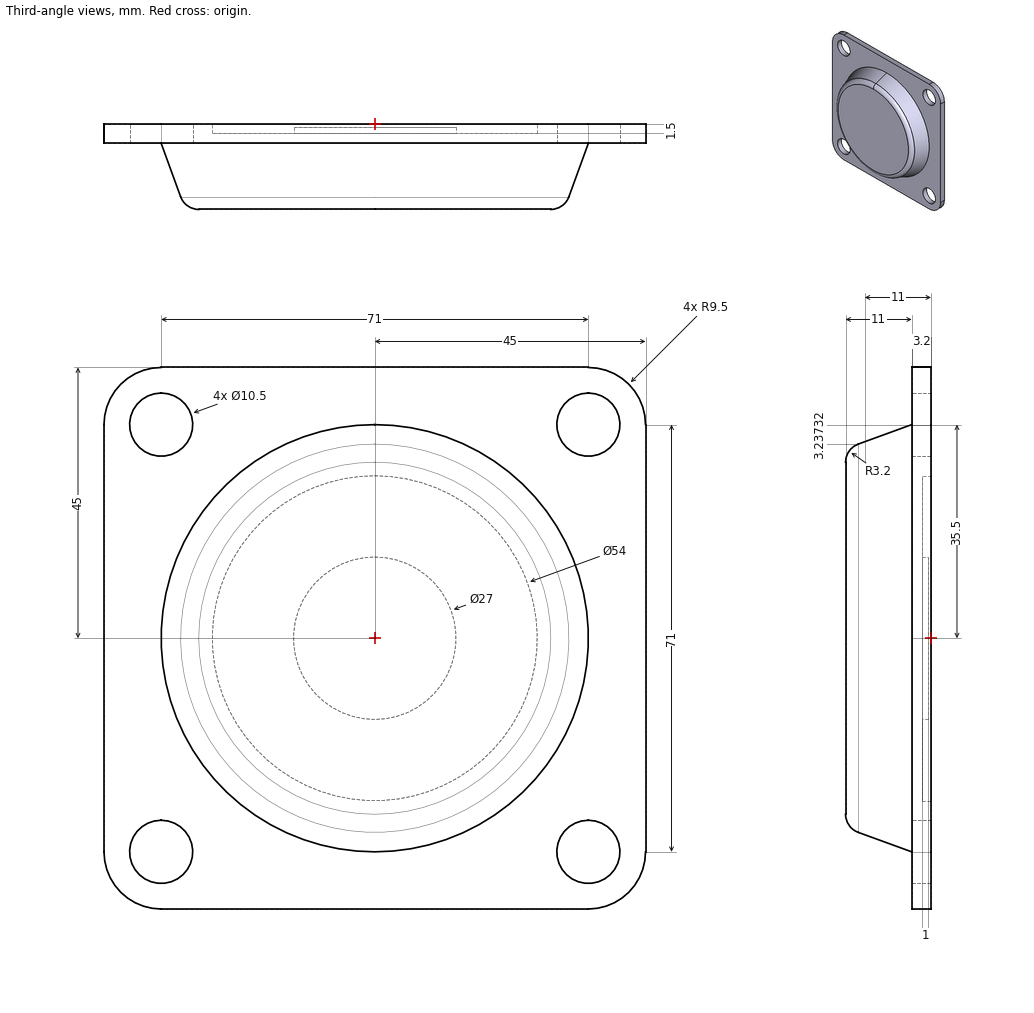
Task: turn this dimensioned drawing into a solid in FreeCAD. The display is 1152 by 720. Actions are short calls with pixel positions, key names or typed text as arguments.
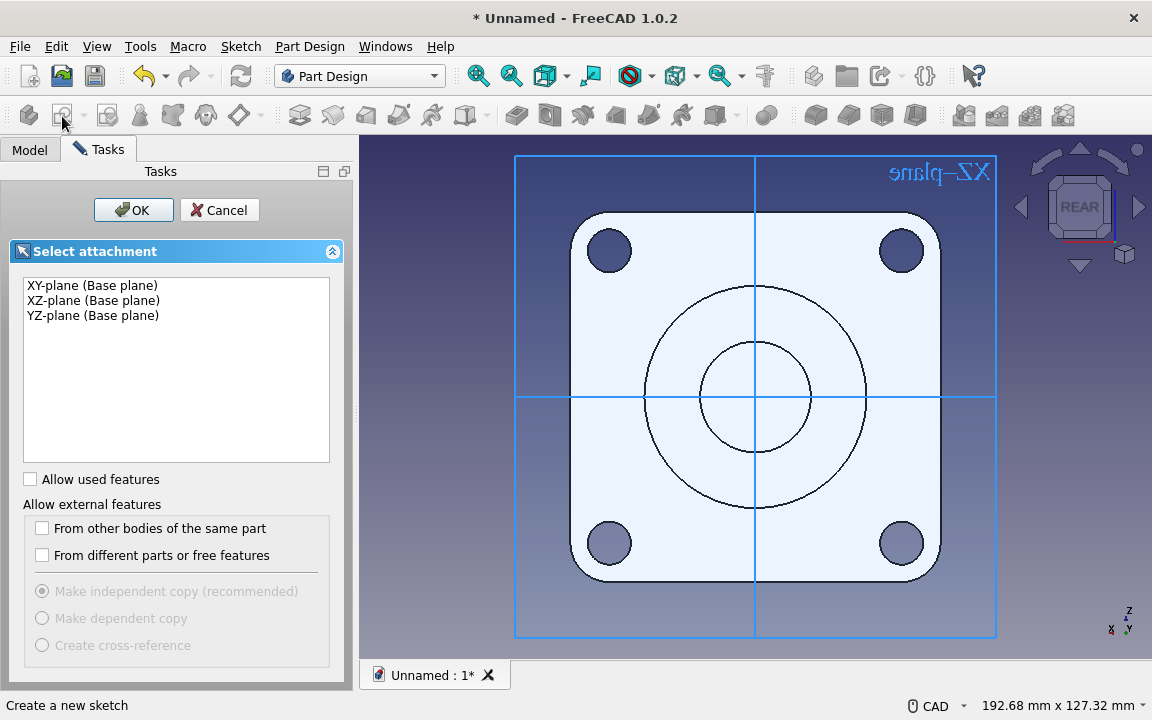
click(84, 316)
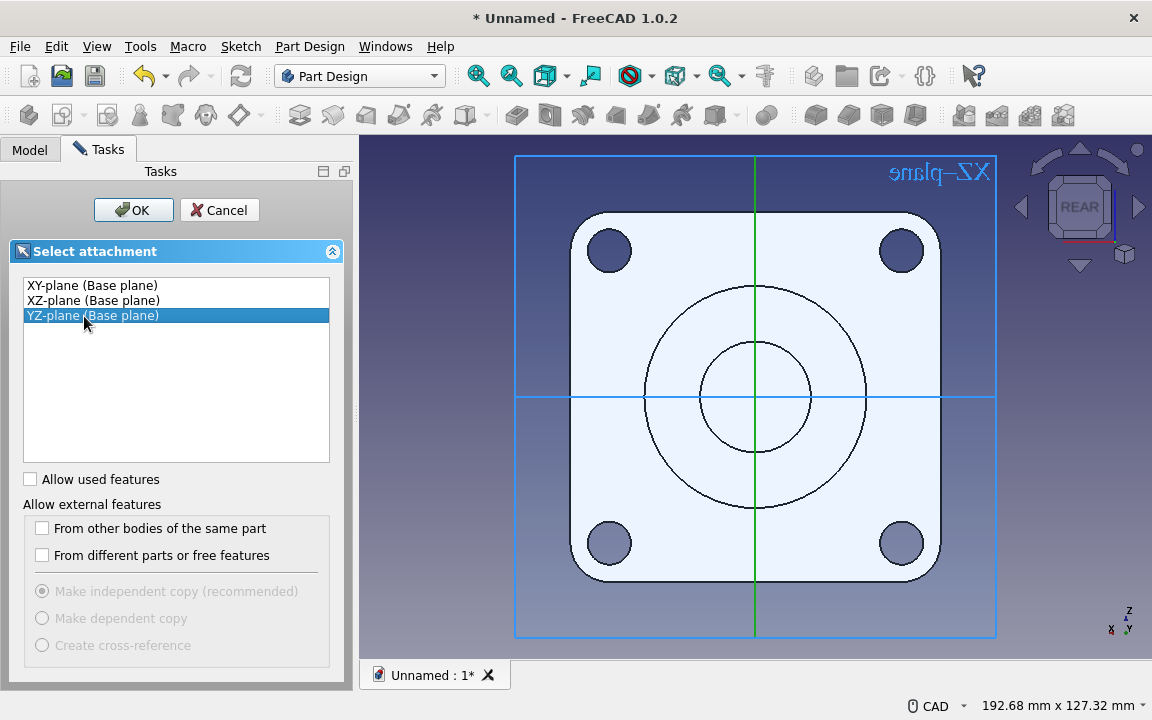
click(134, 210)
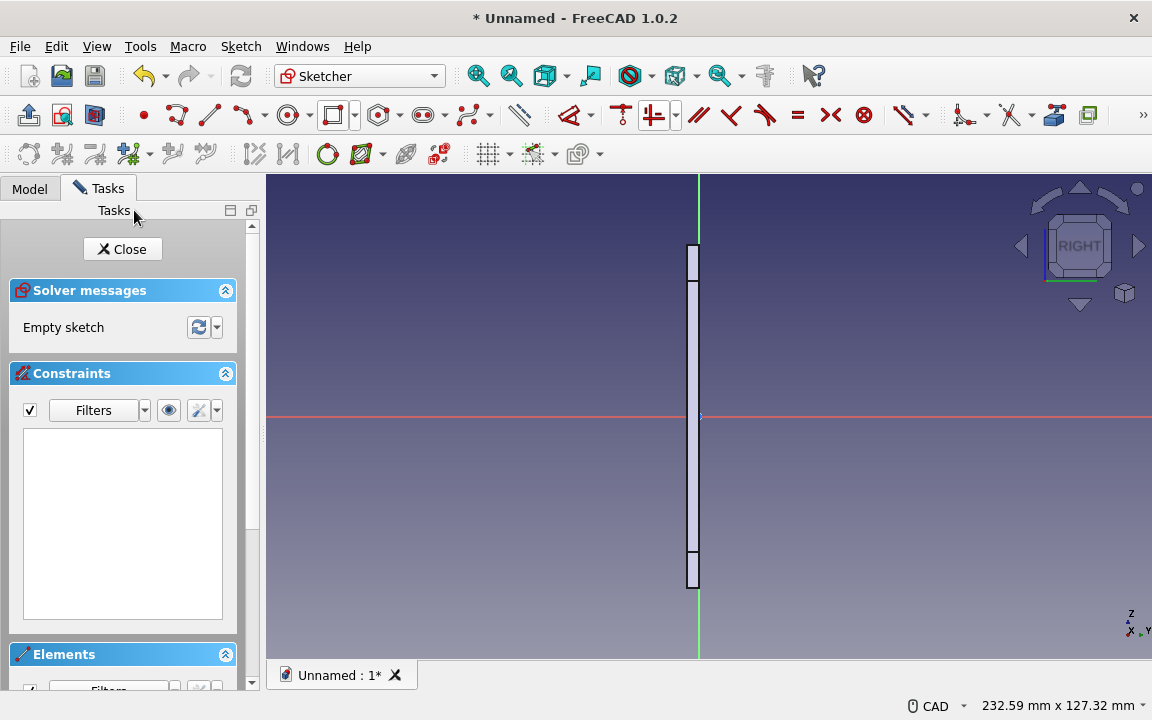
click(95, 116)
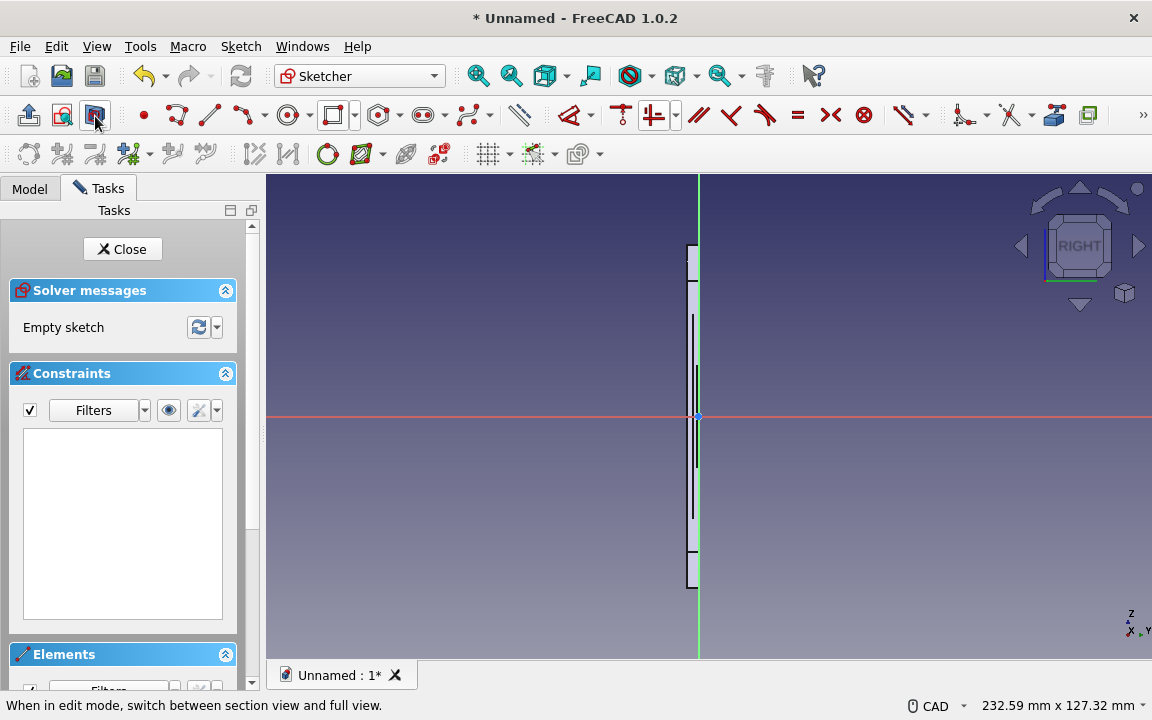
scroll(697, 294, up, 4)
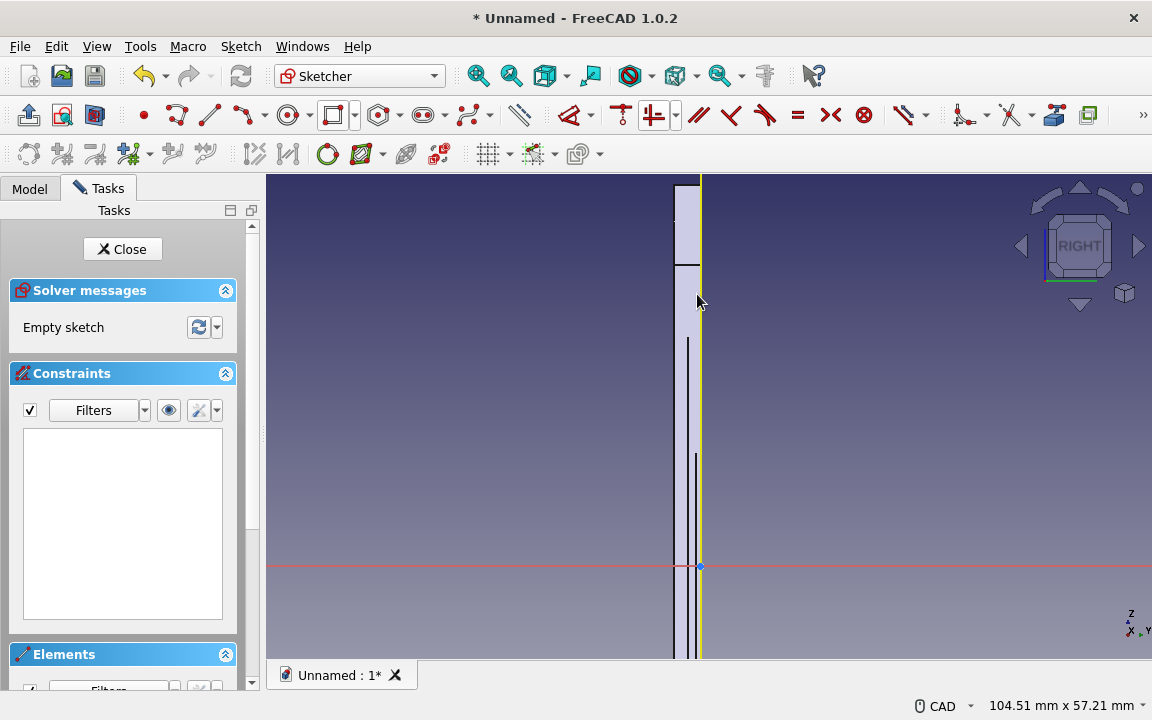
key(g)
key(m)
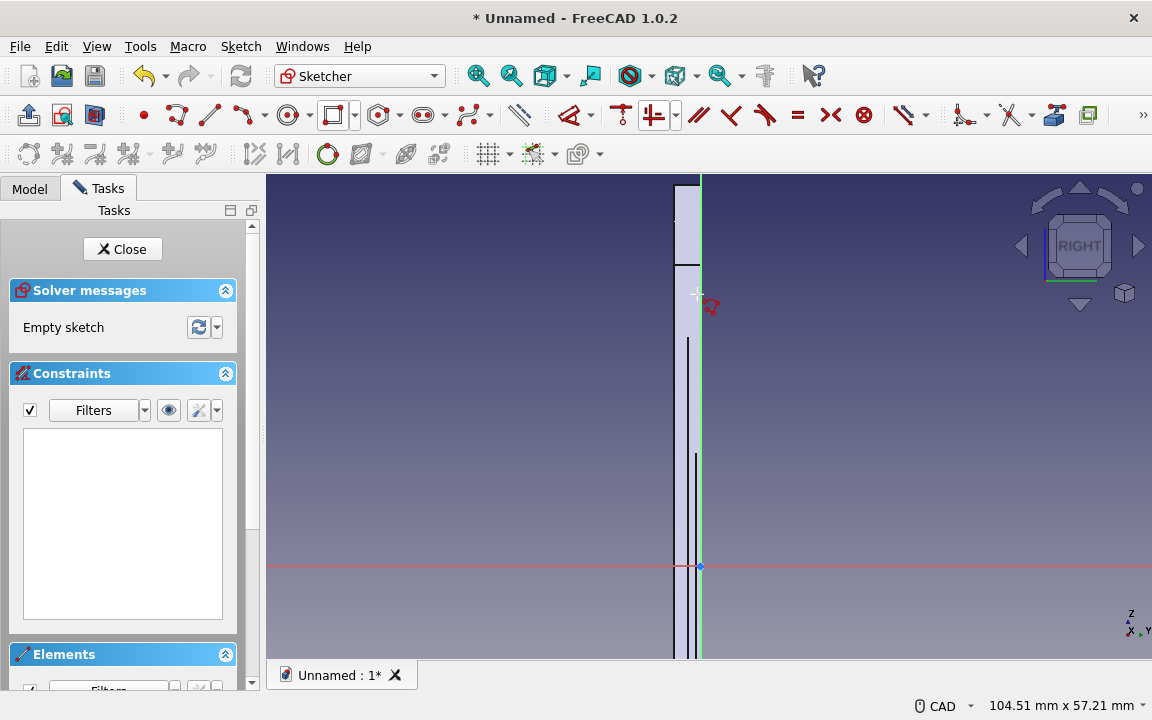
click(580, 318)
click(580, 566)
click(674, 557)
click(674, 265)
click(598, 293)
right_click(598, 293)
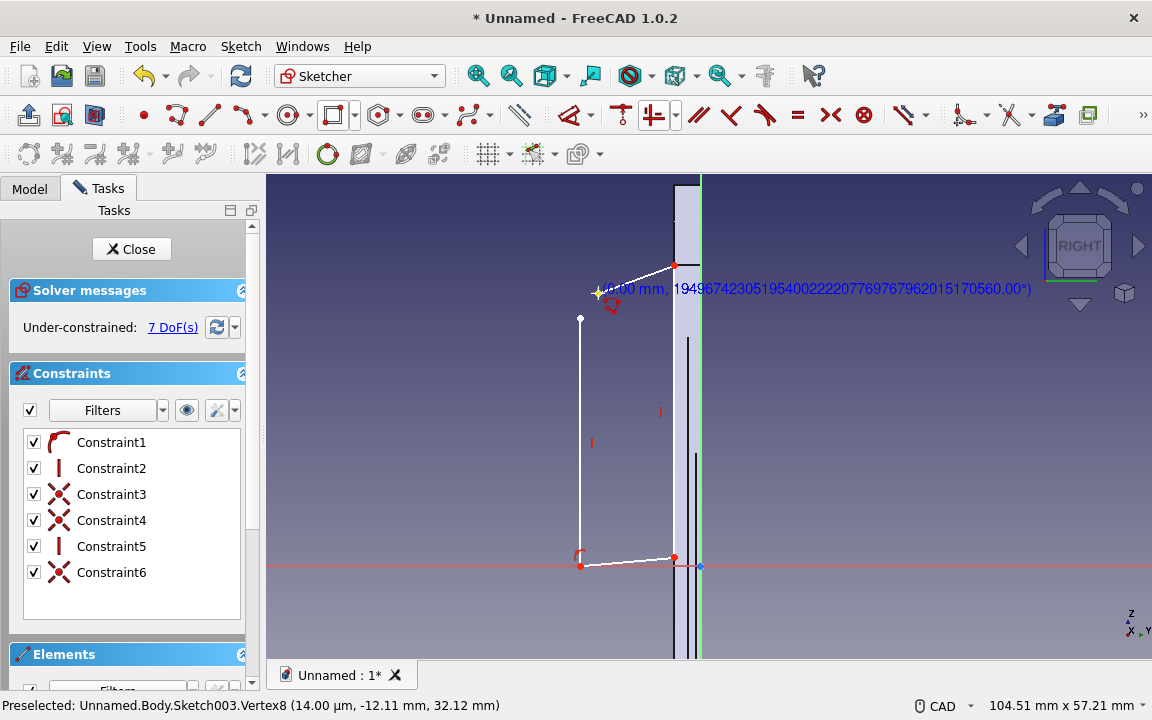
key(g)
key(3)
key(a)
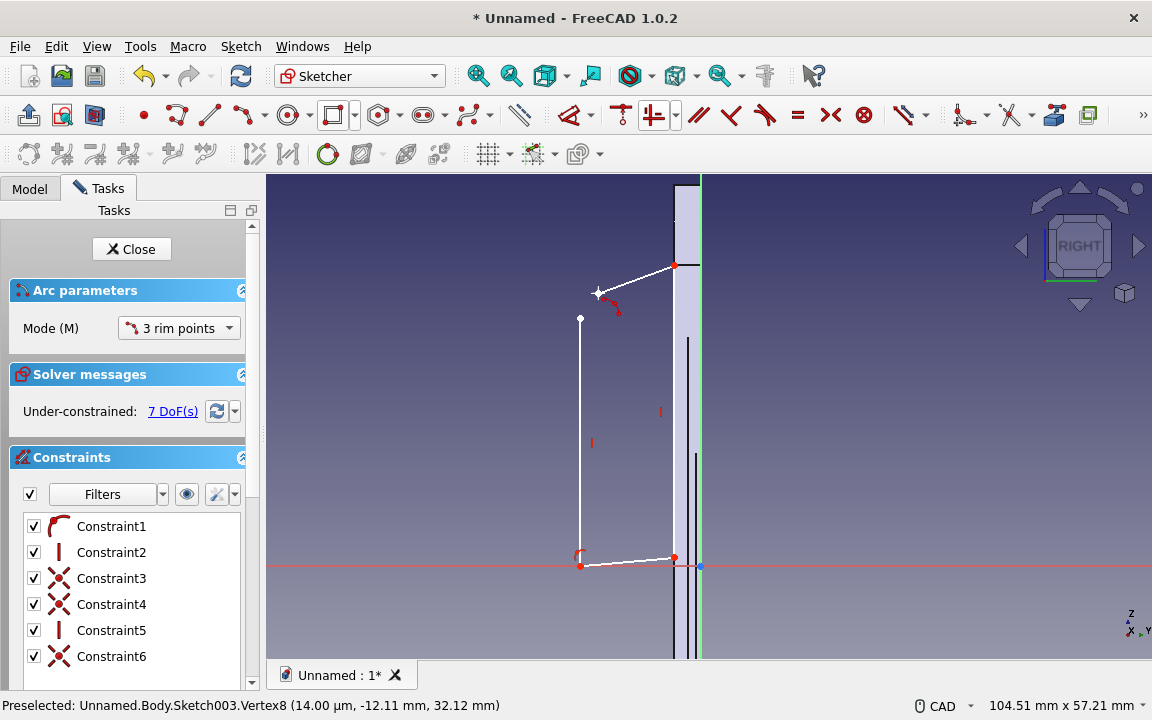
click(598, 294)
click(580, 319)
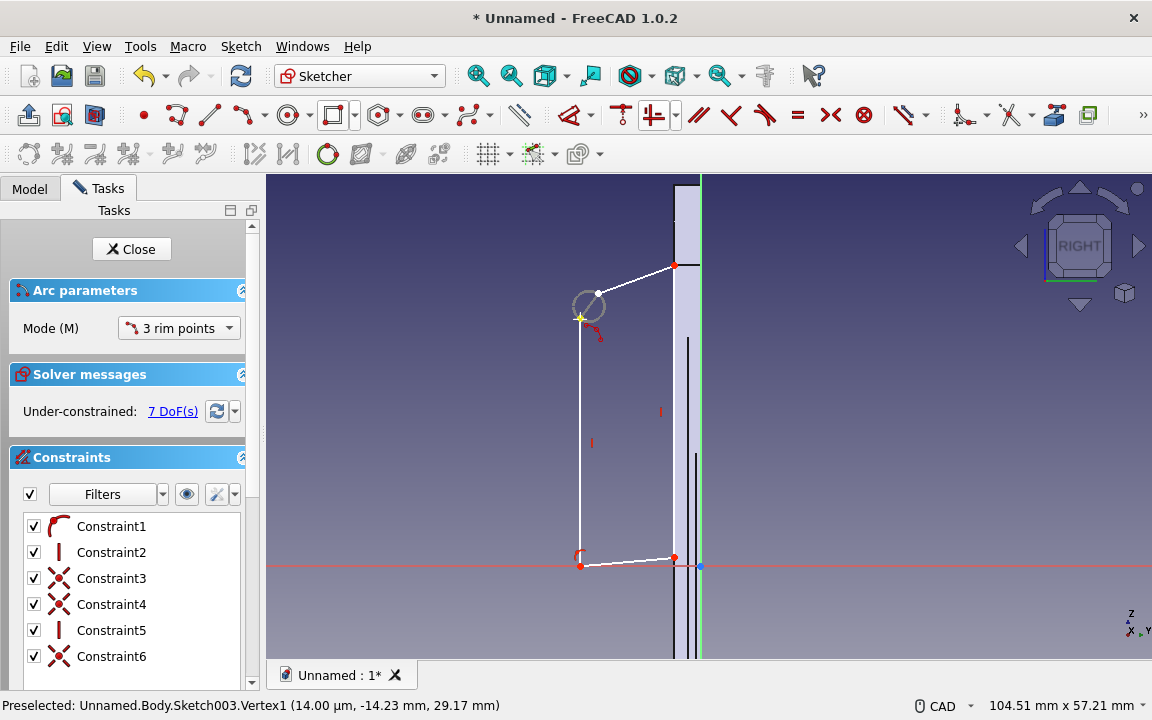
scroll(585, 303, up, 6)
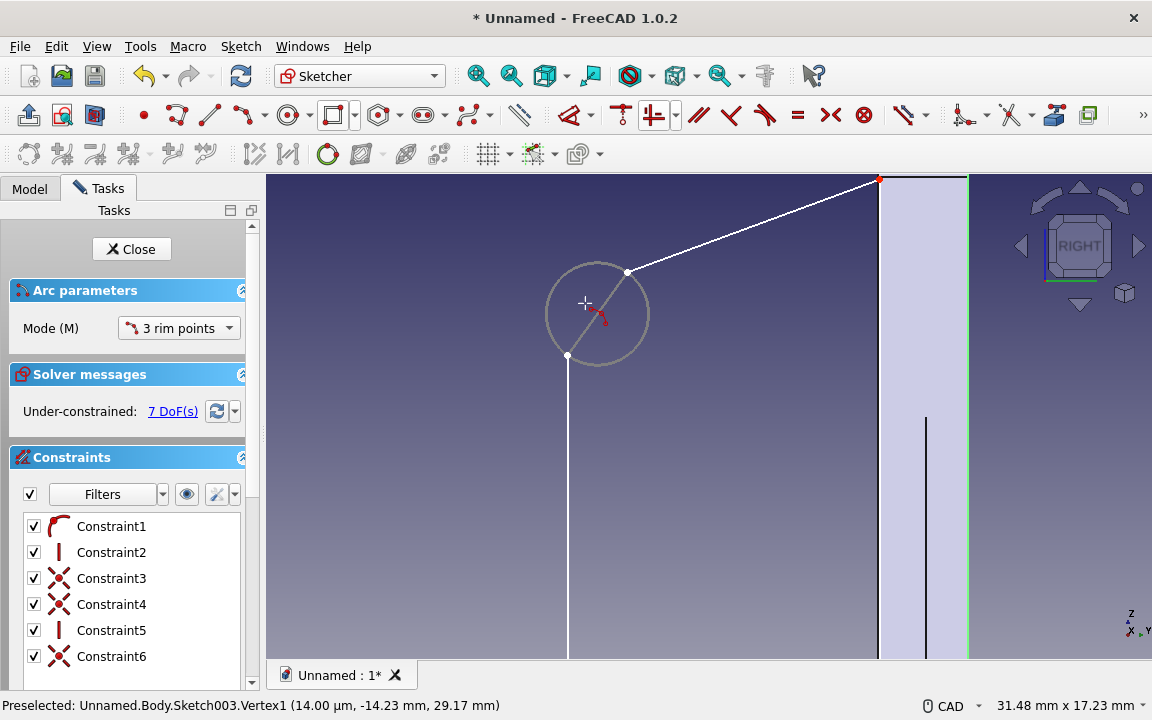
click(585, 302)
key(Escape)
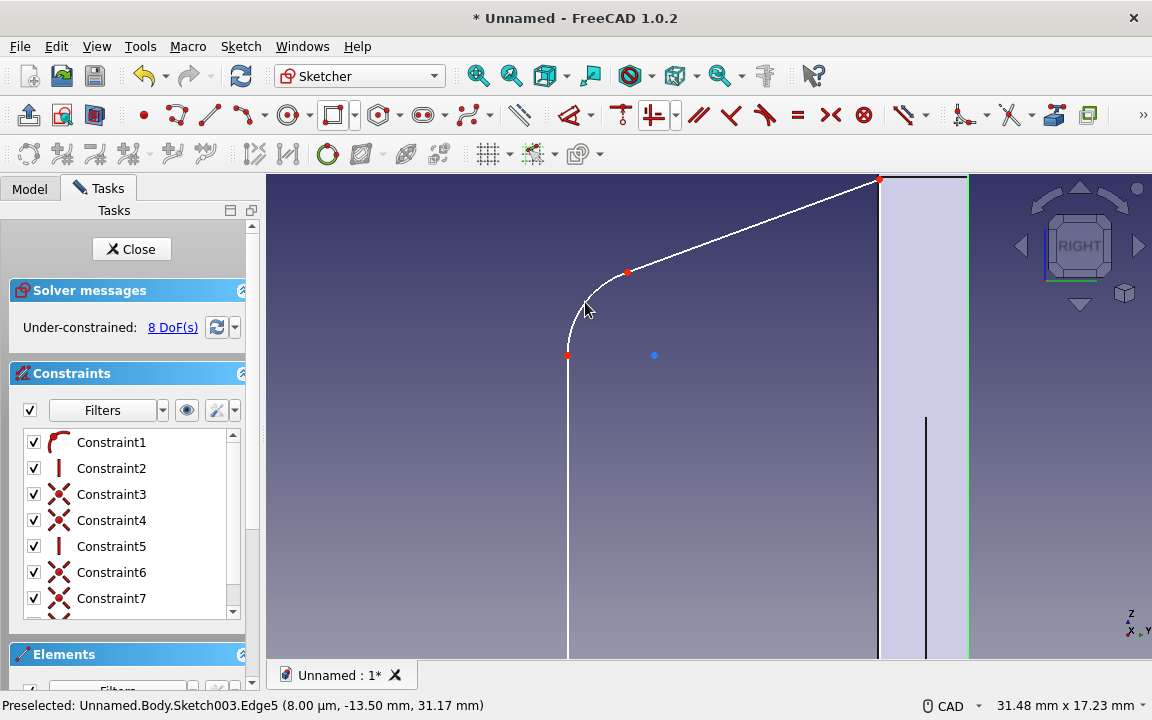
click(568, 602)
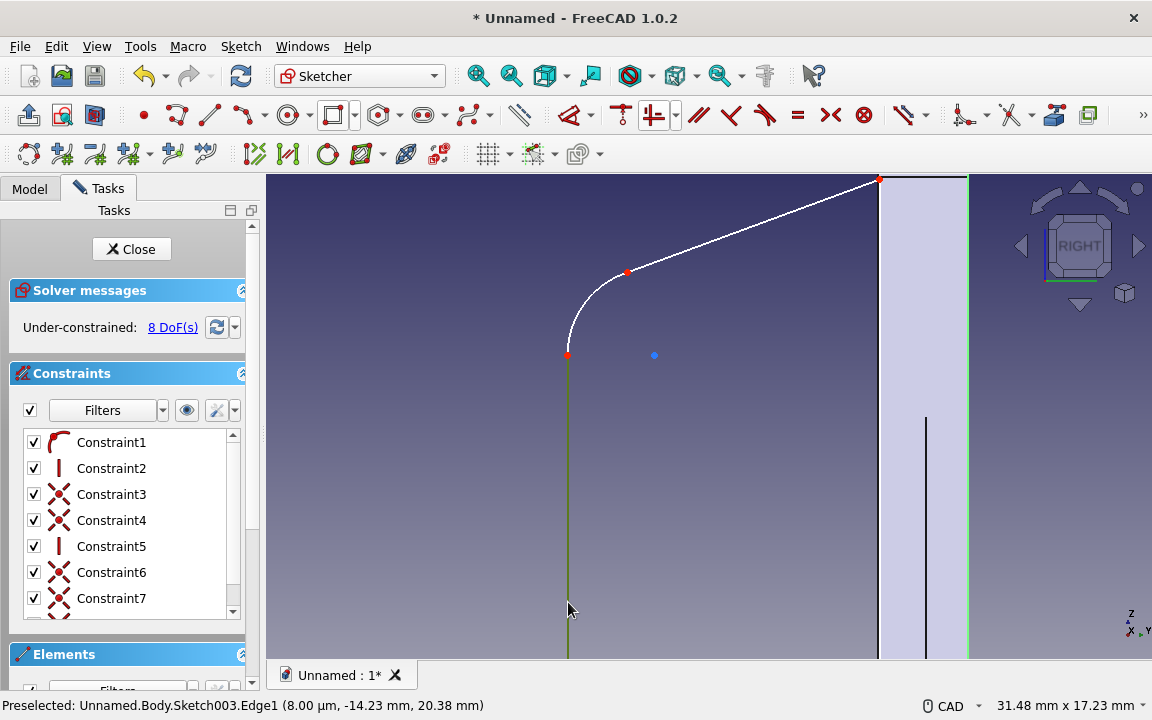
click(599, 288)